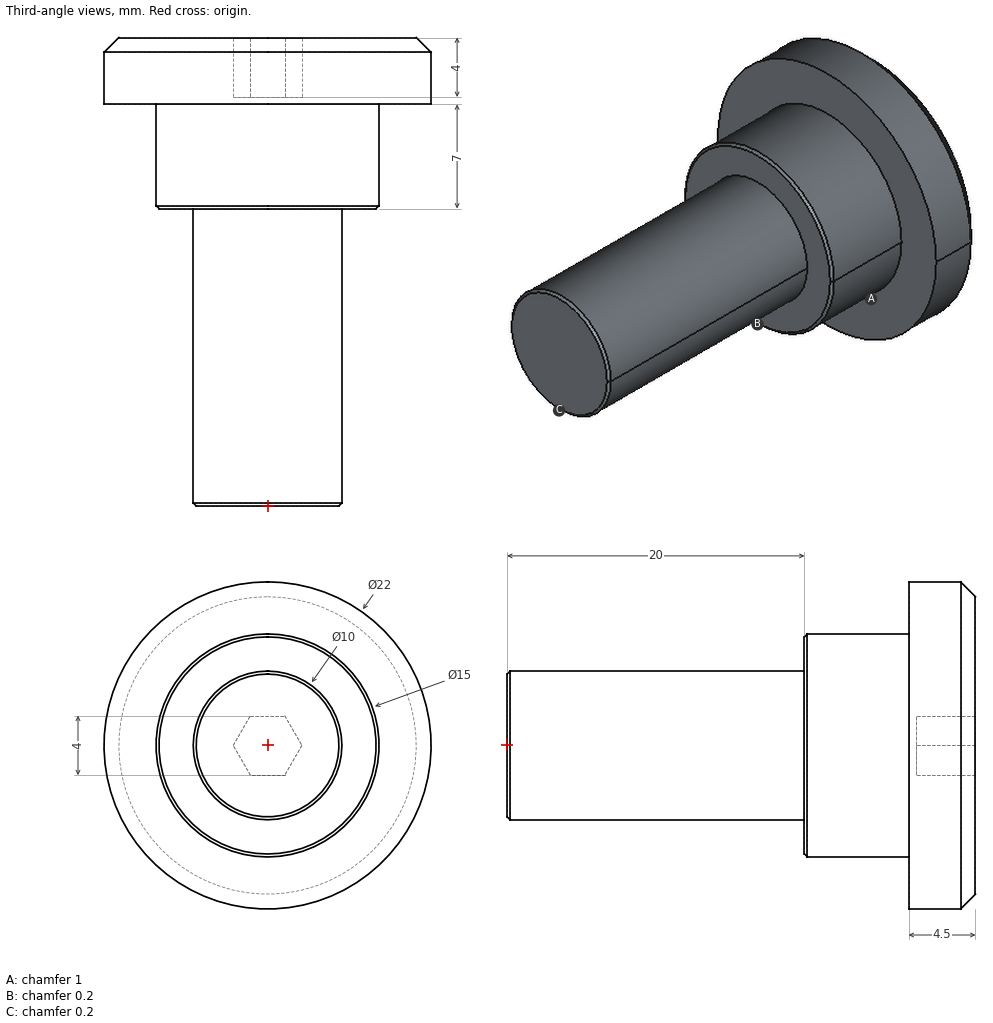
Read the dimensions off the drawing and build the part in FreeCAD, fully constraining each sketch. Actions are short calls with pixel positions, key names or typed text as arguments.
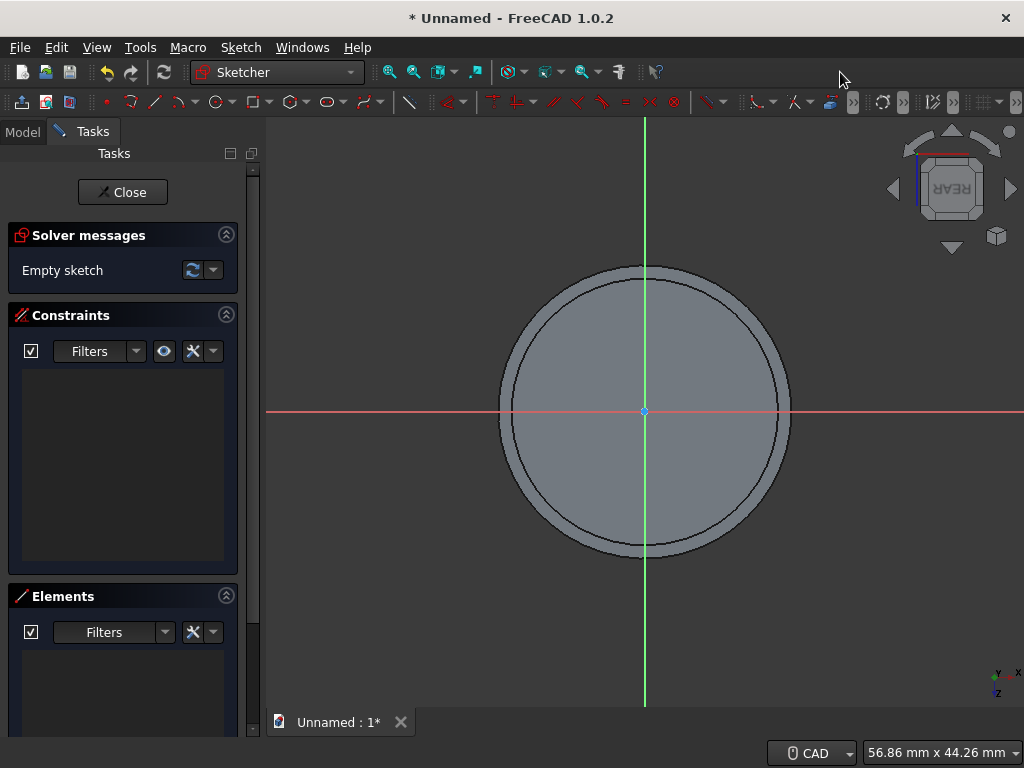
scroll(658, 412, up, 9)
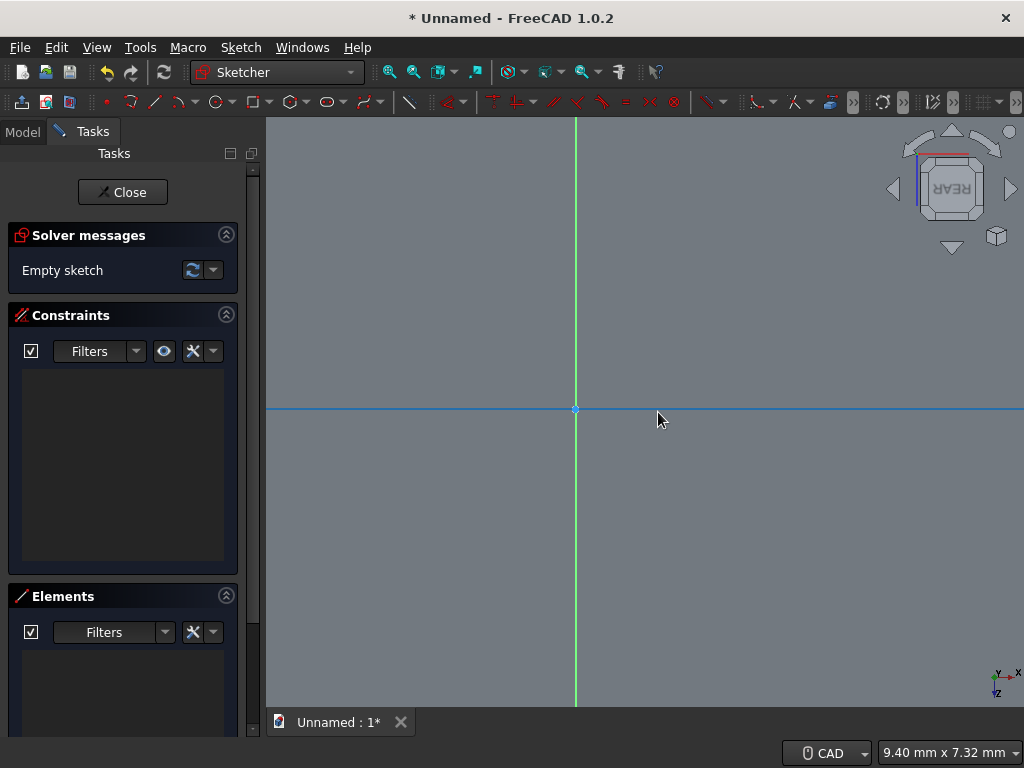
click(290, 102)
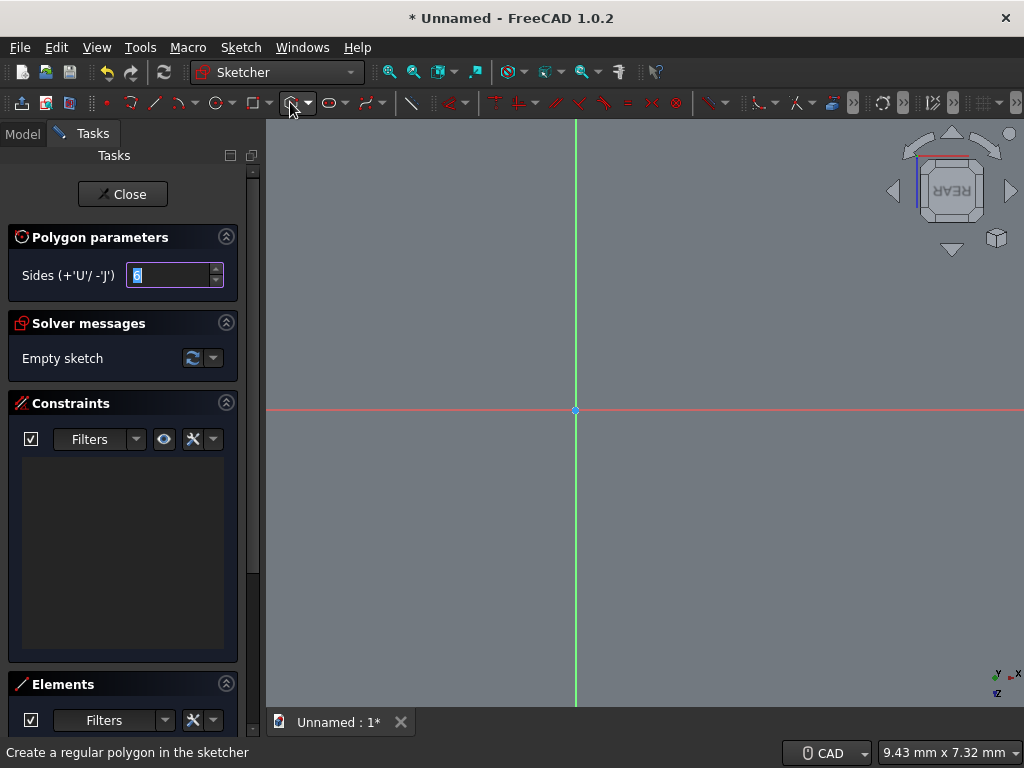
click(576, 410)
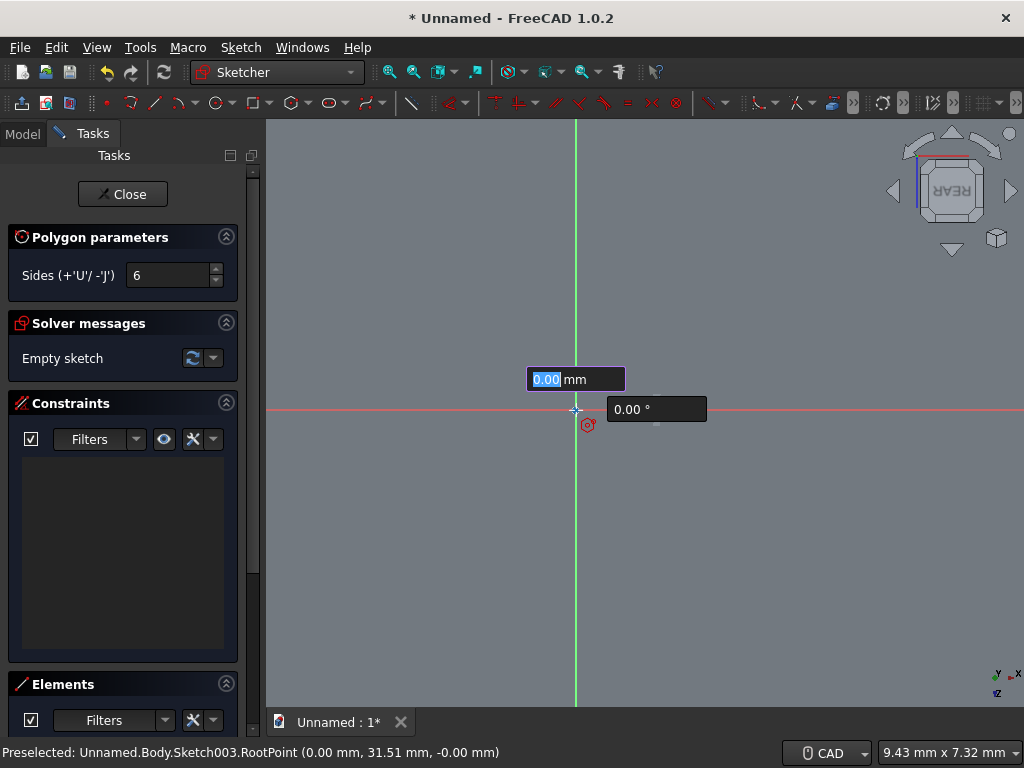
click(762, 410)
key(Escape)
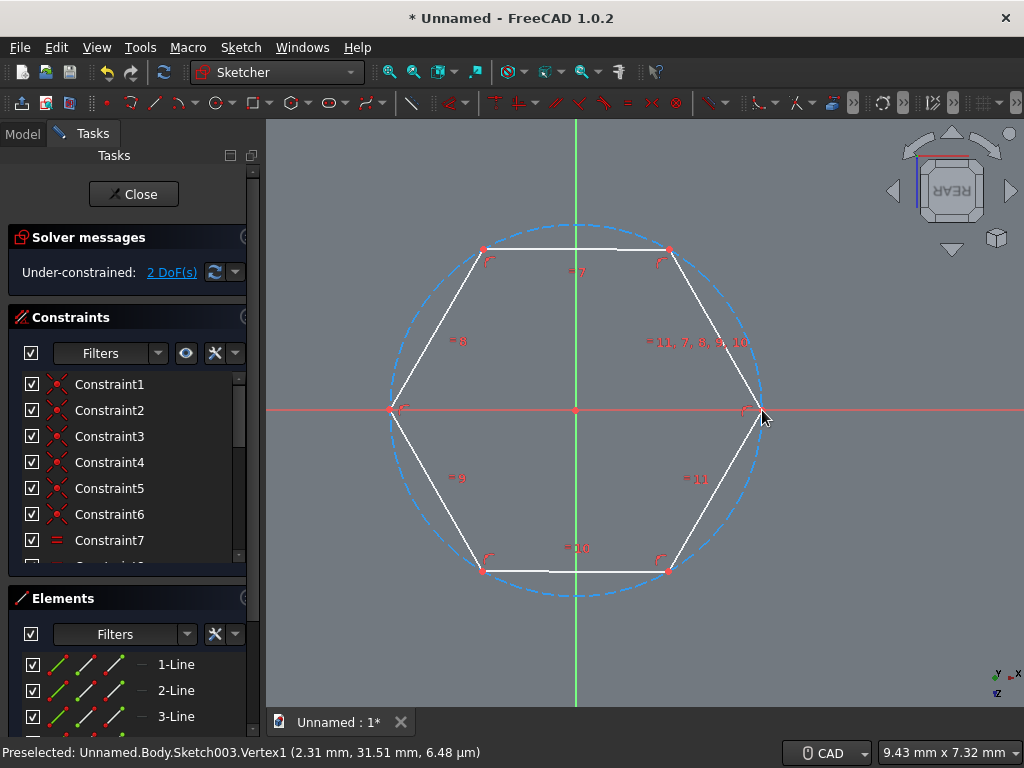
click(614, 249)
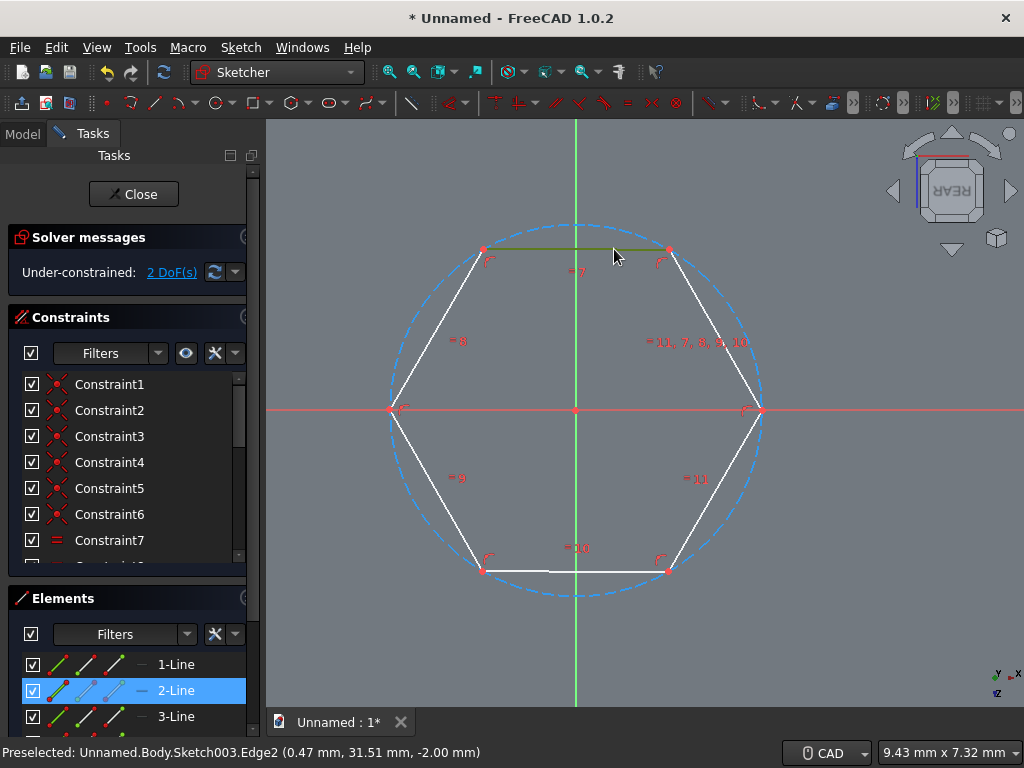
key(h)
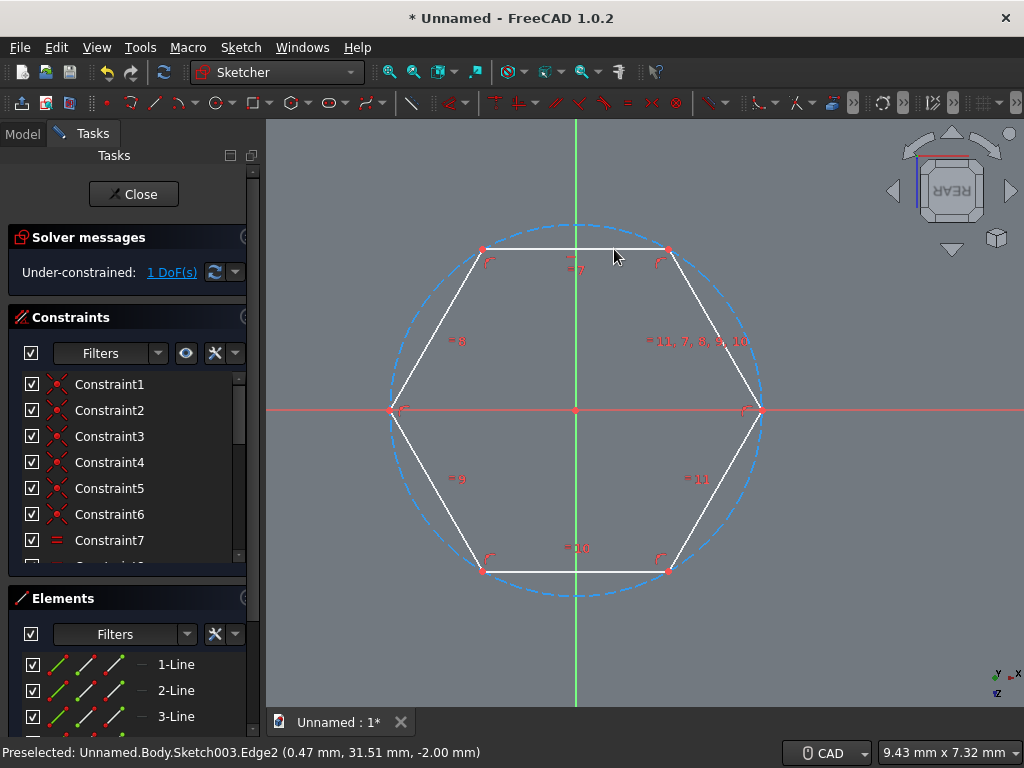
key(d)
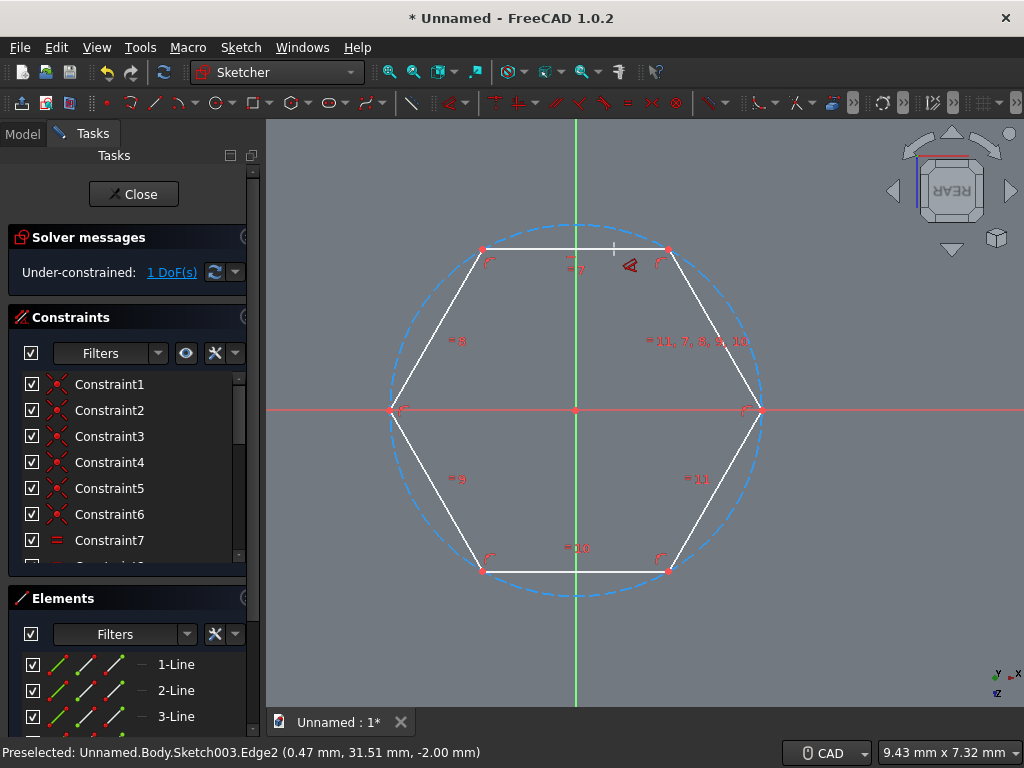
click(483, 572)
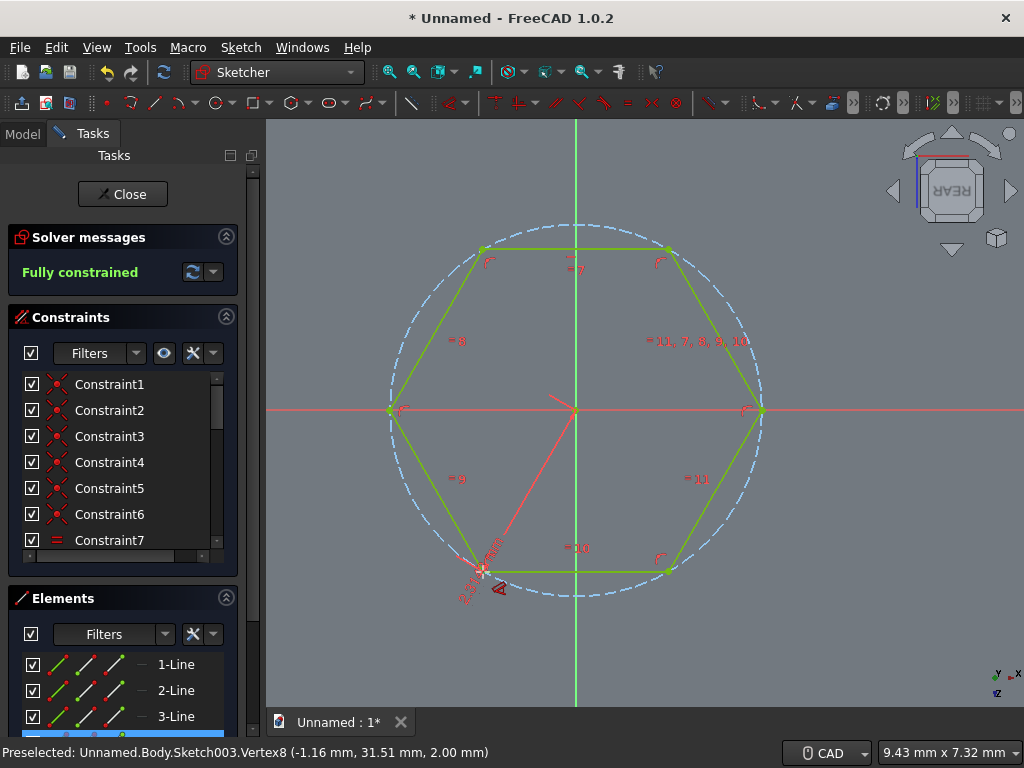
click(669, 249)
click(703, 336)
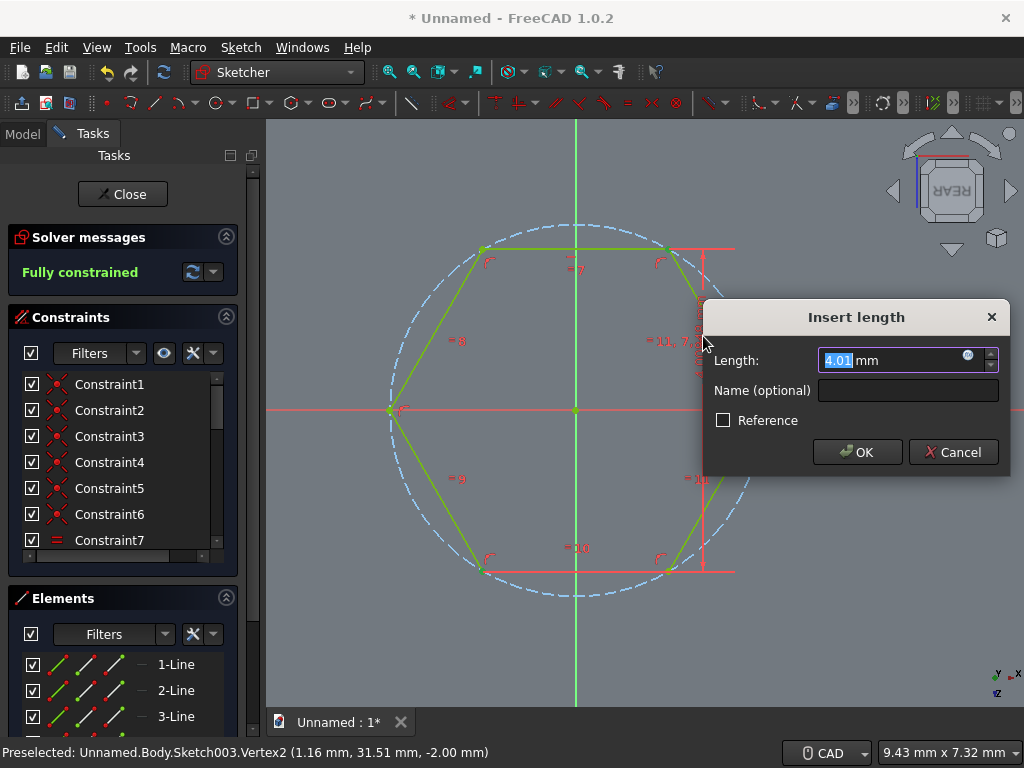
text(4)
key(Return)
key(Escape)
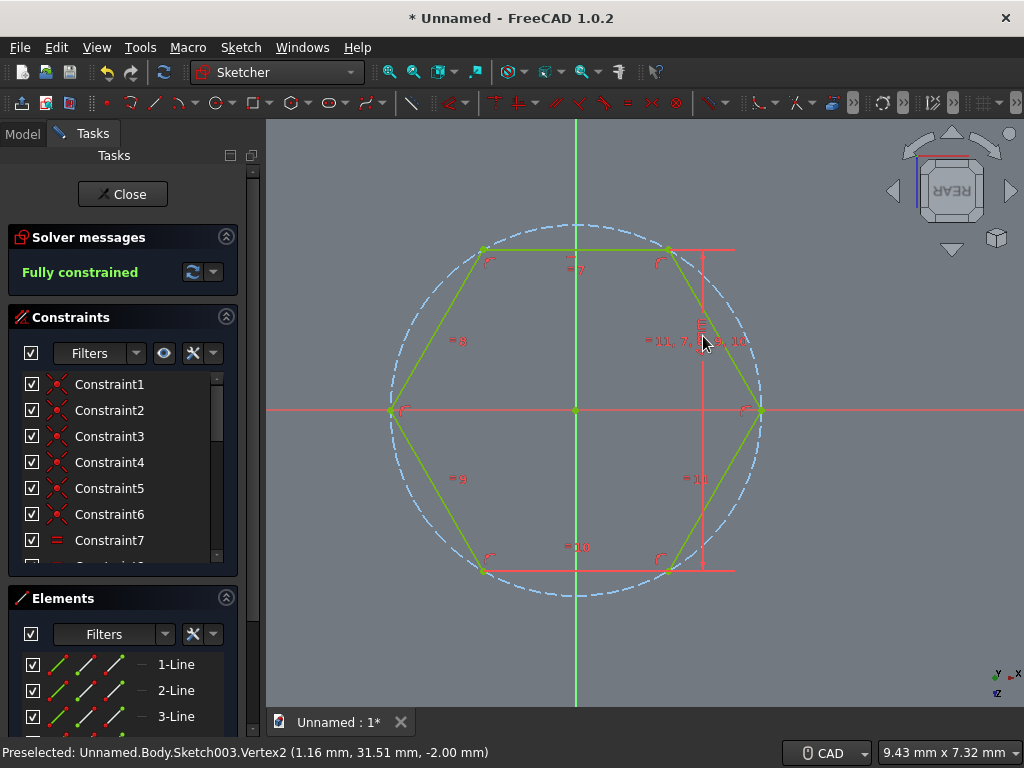
click(123, 194)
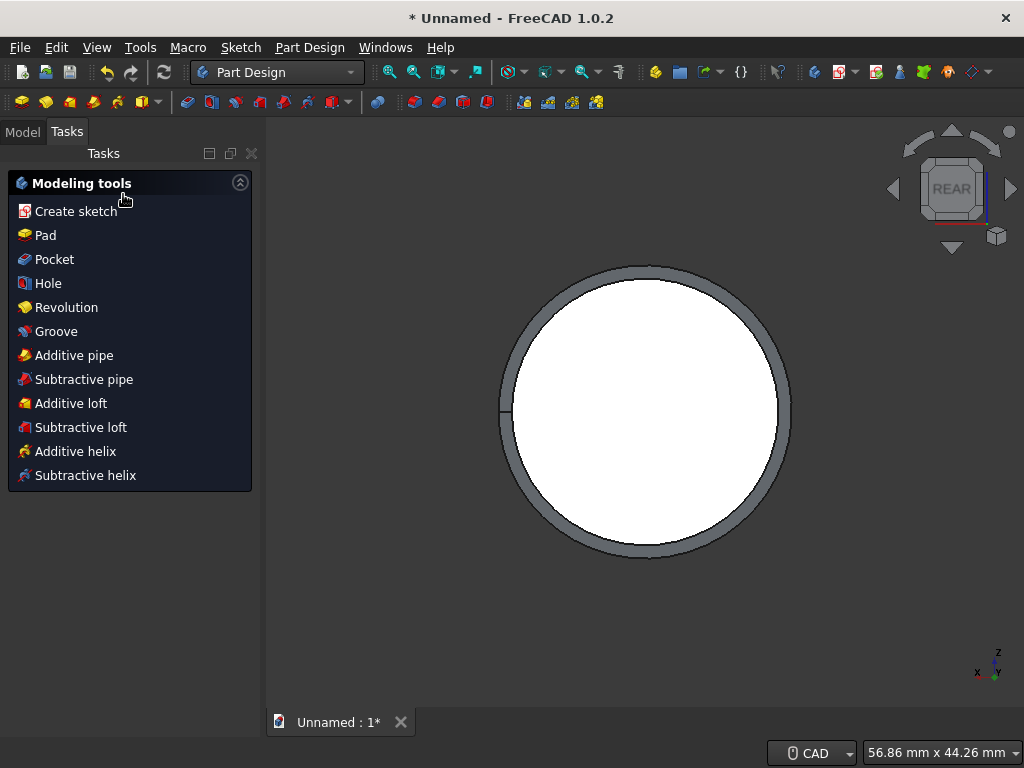
click(188, 102)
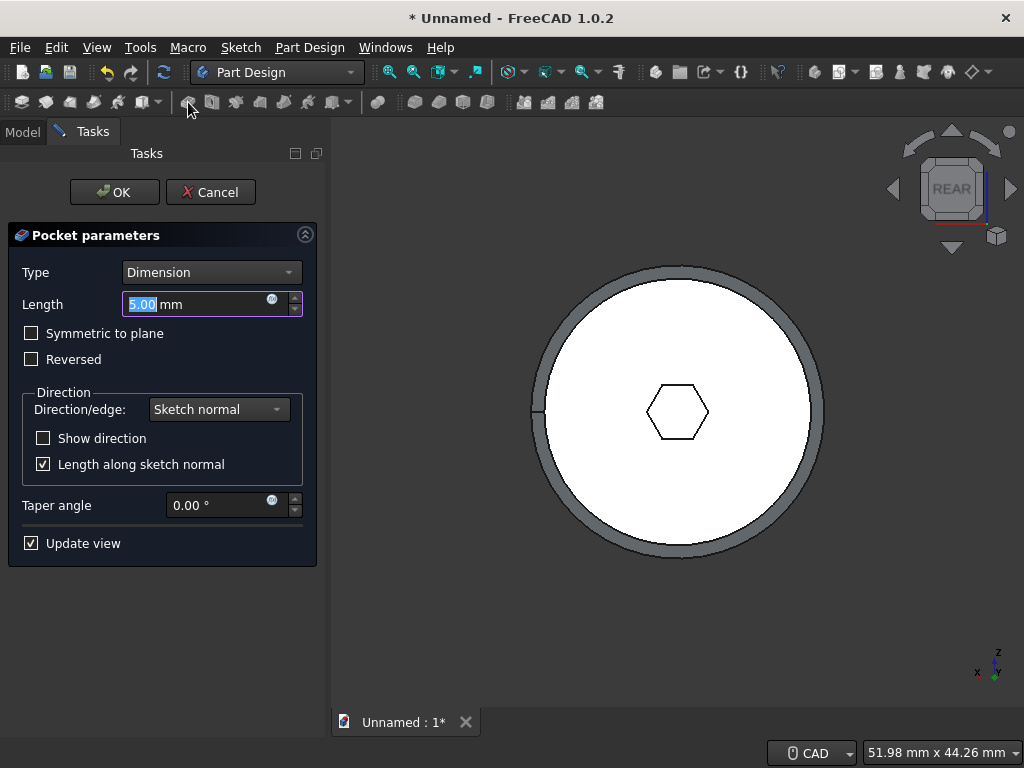
text(4)
key(Tab)